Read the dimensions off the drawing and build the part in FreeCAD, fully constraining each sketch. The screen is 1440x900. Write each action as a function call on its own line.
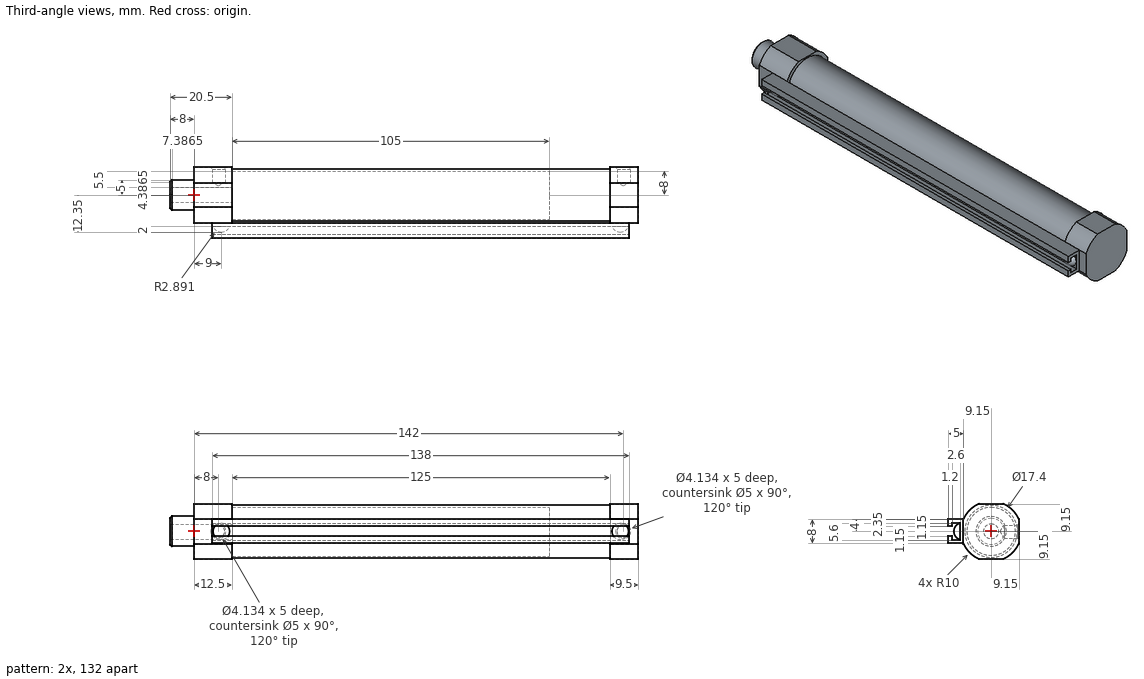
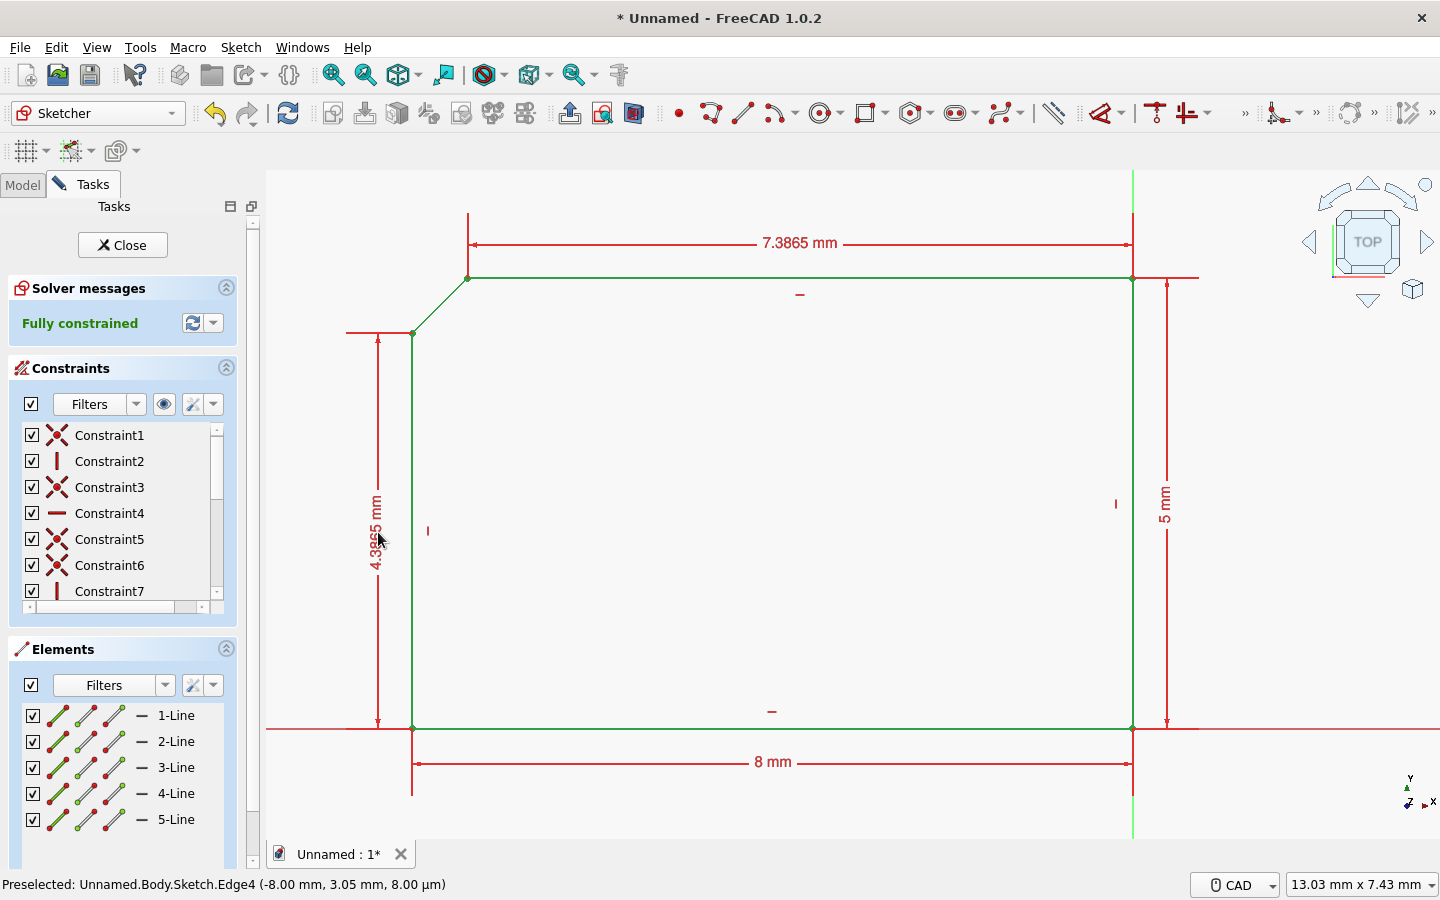
click(123, 245)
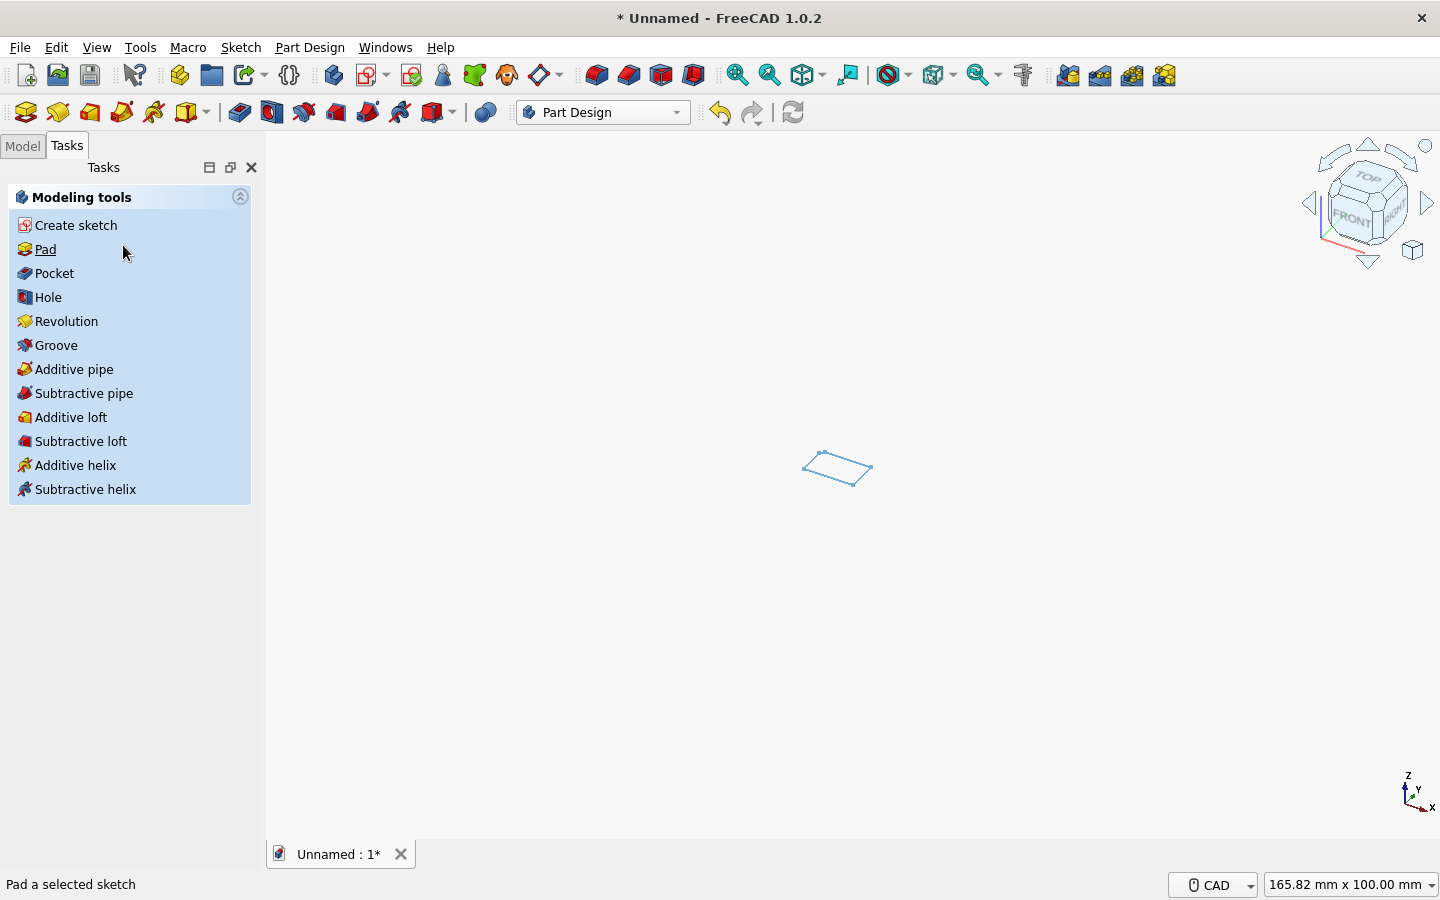
click(58, 112)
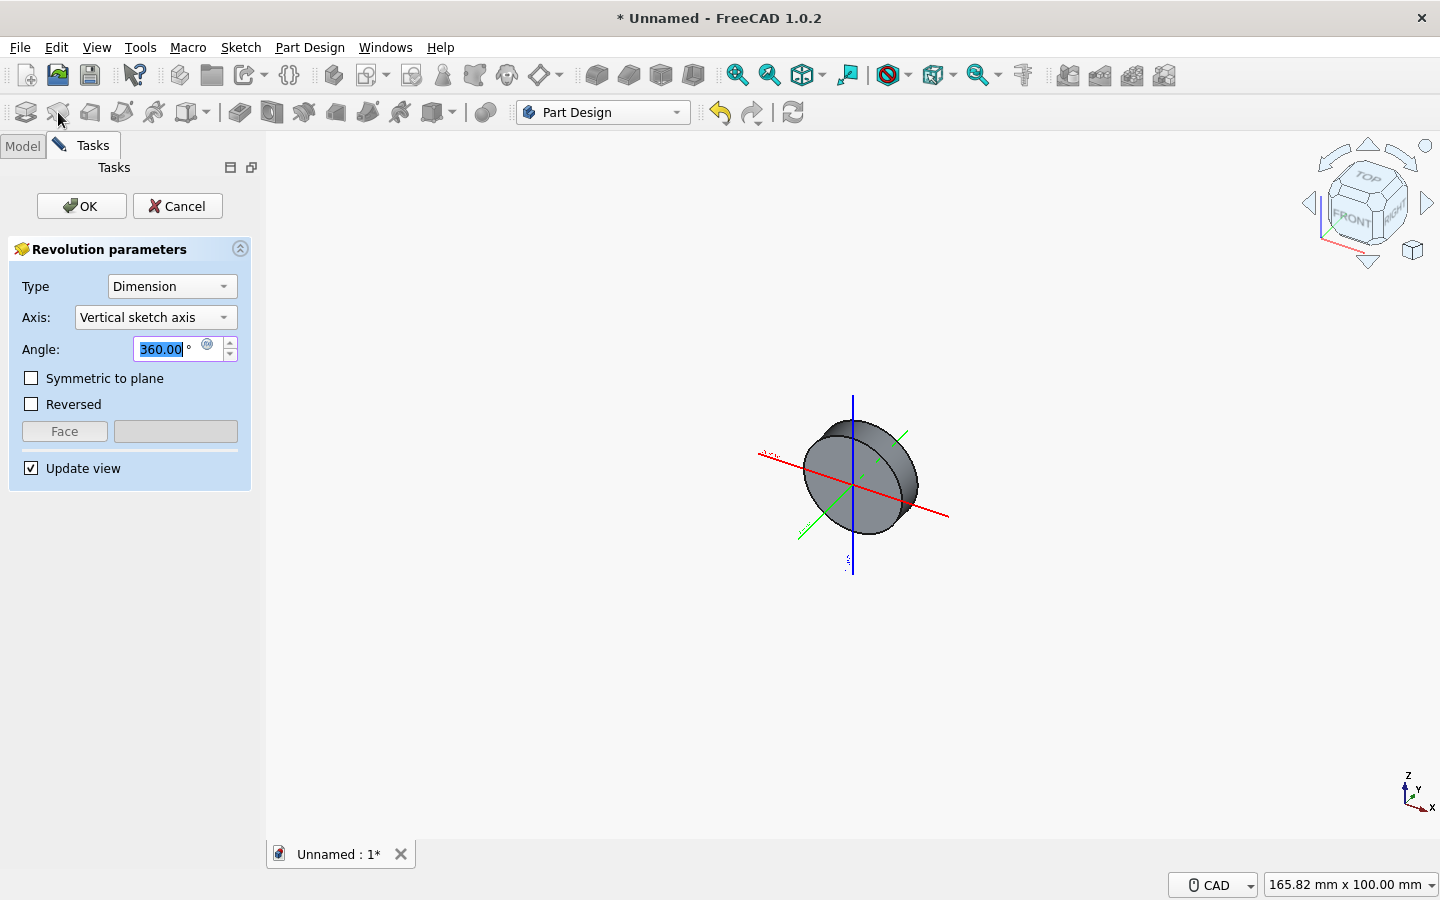
click(156, 318)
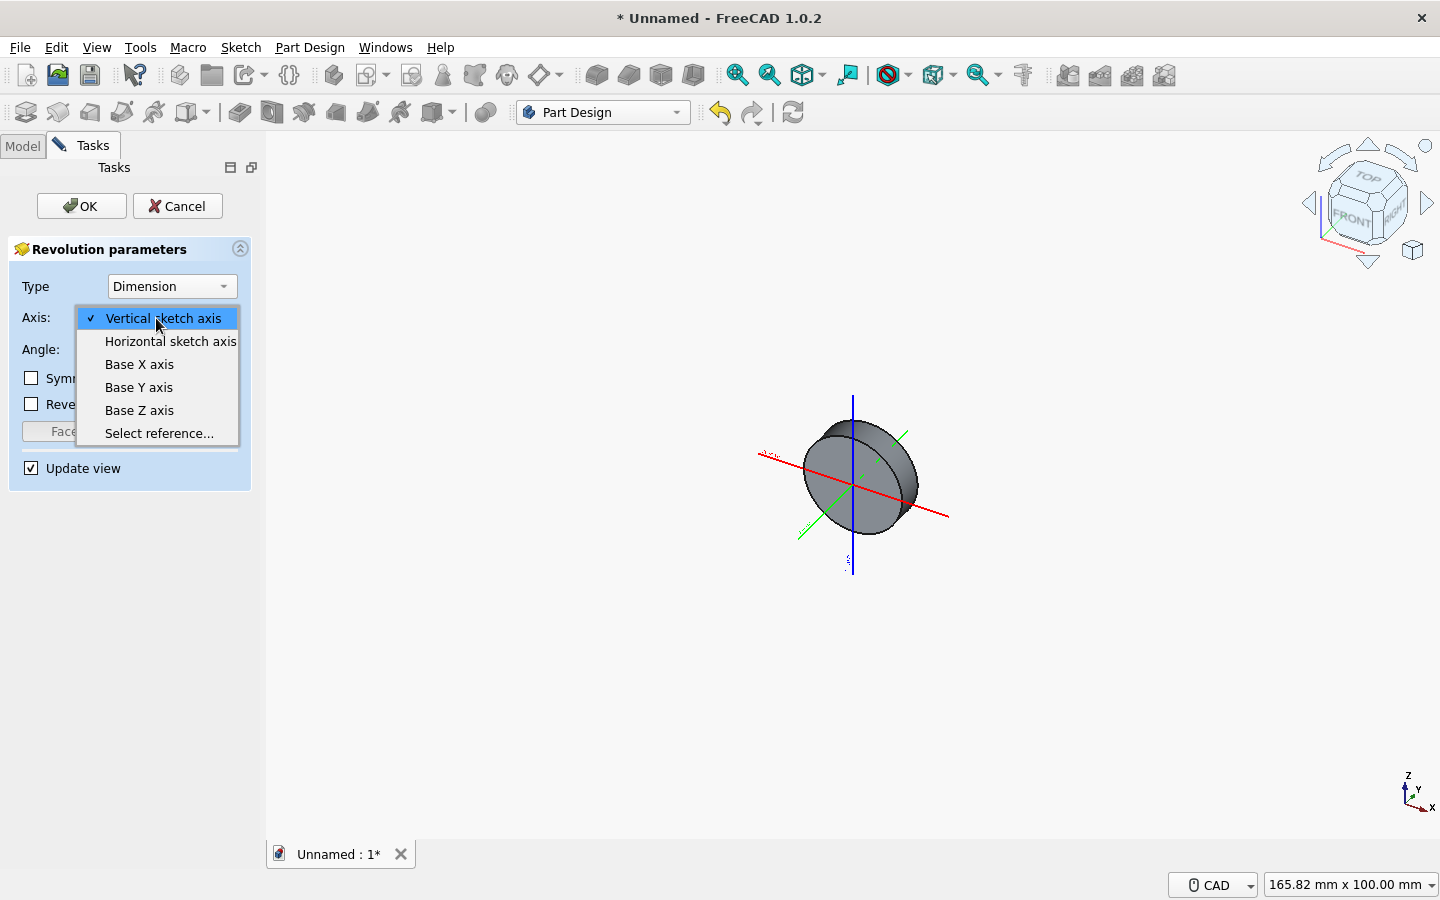
click(156, 342)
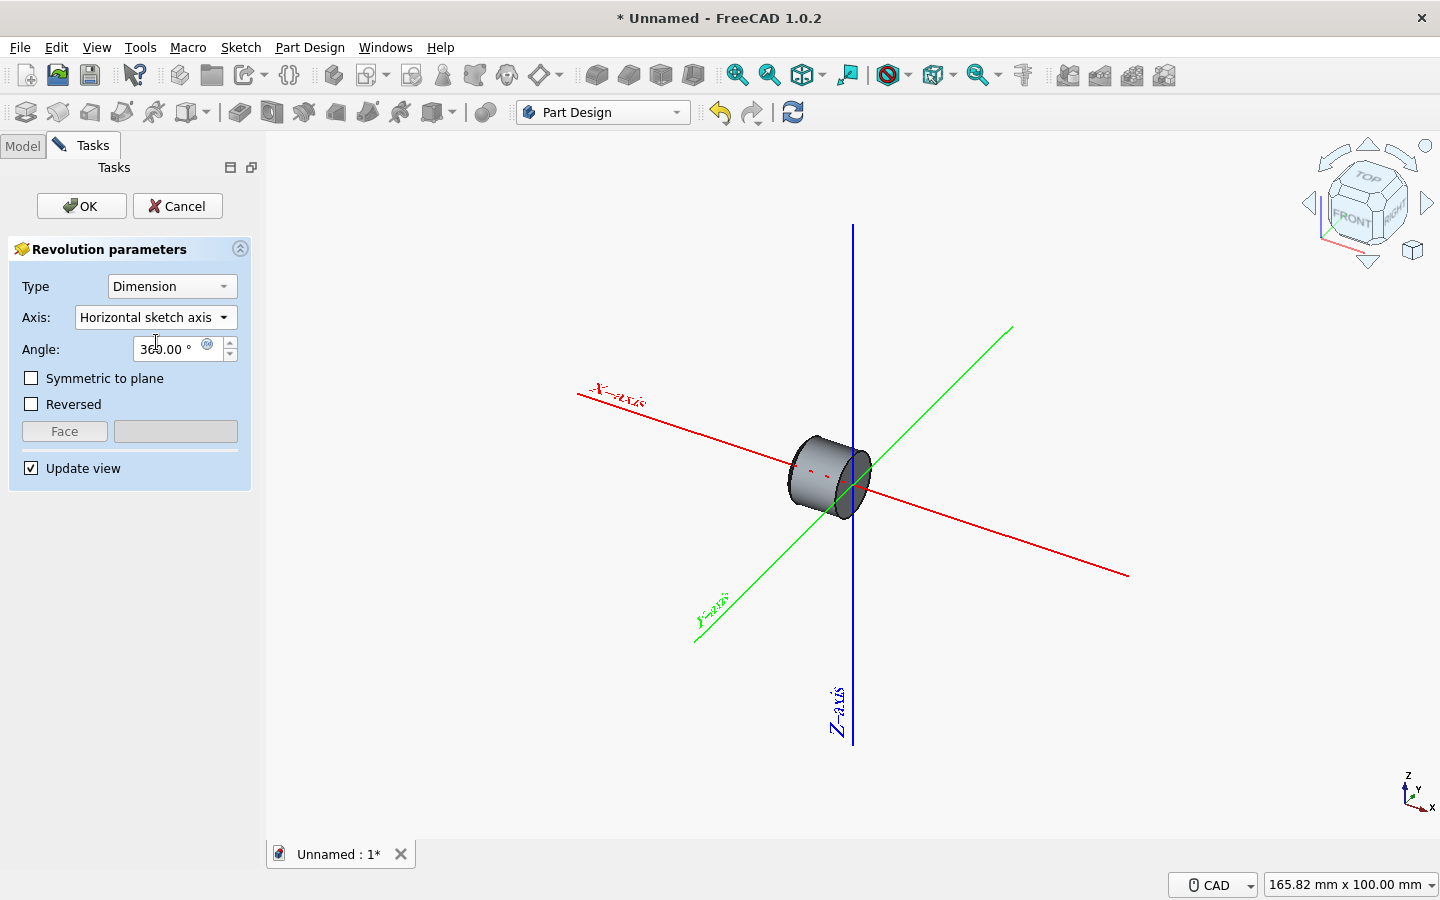
click(82, 206)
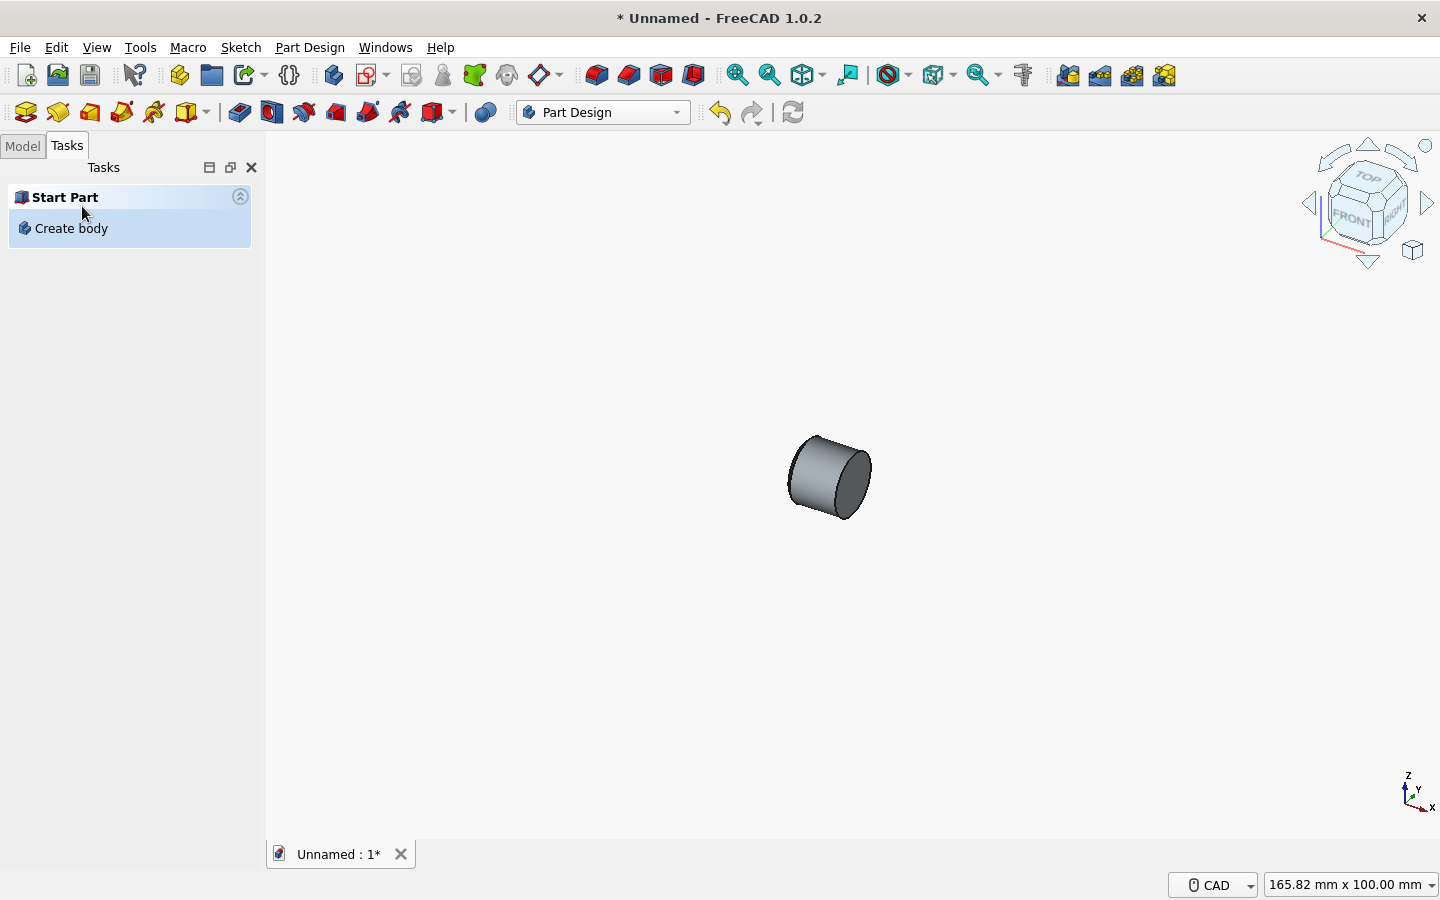
click(738, 76)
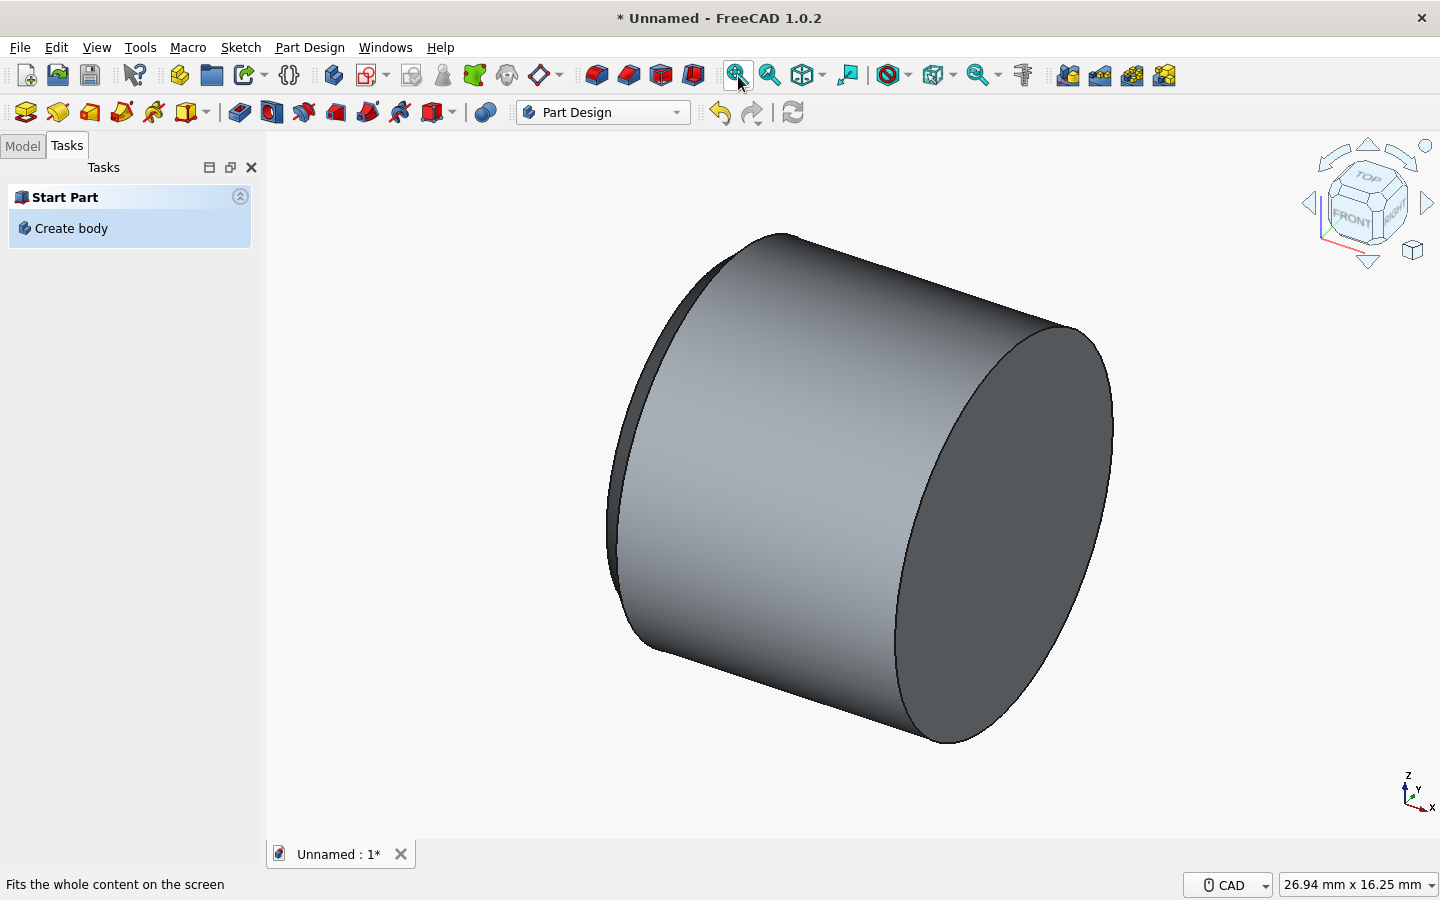
click(1004, 534)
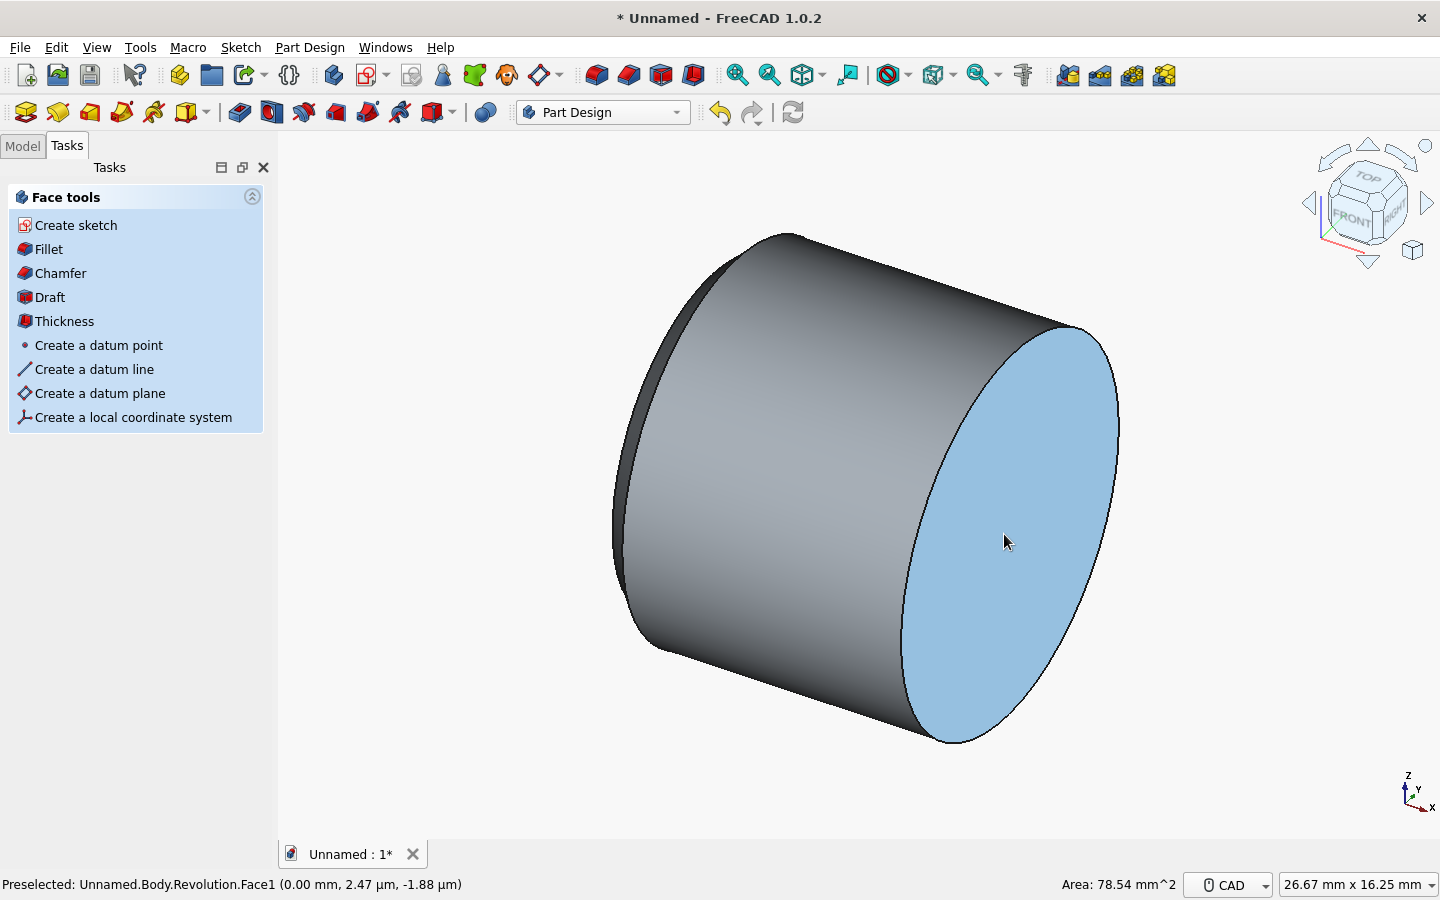
click(366, 76)